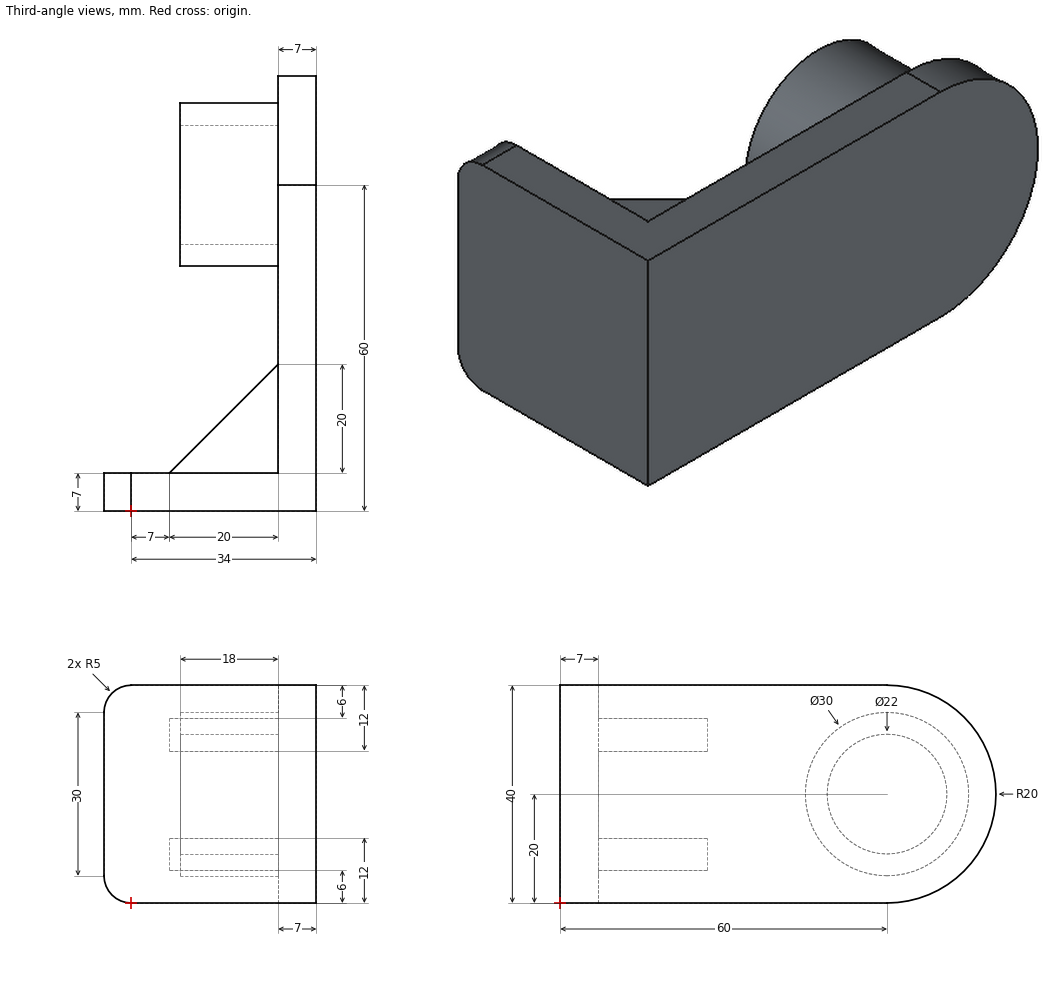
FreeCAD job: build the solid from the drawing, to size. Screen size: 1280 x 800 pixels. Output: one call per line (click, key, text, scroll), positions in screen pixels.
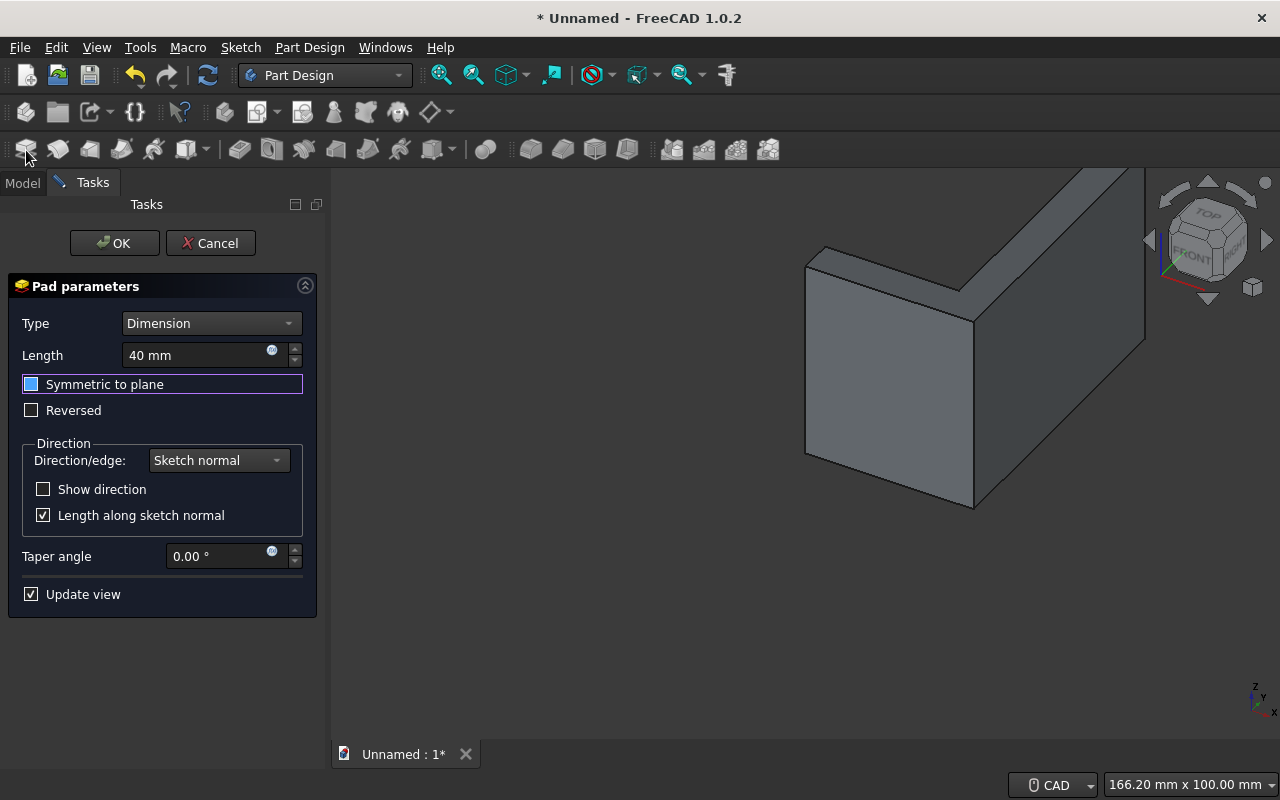
click(115, 243)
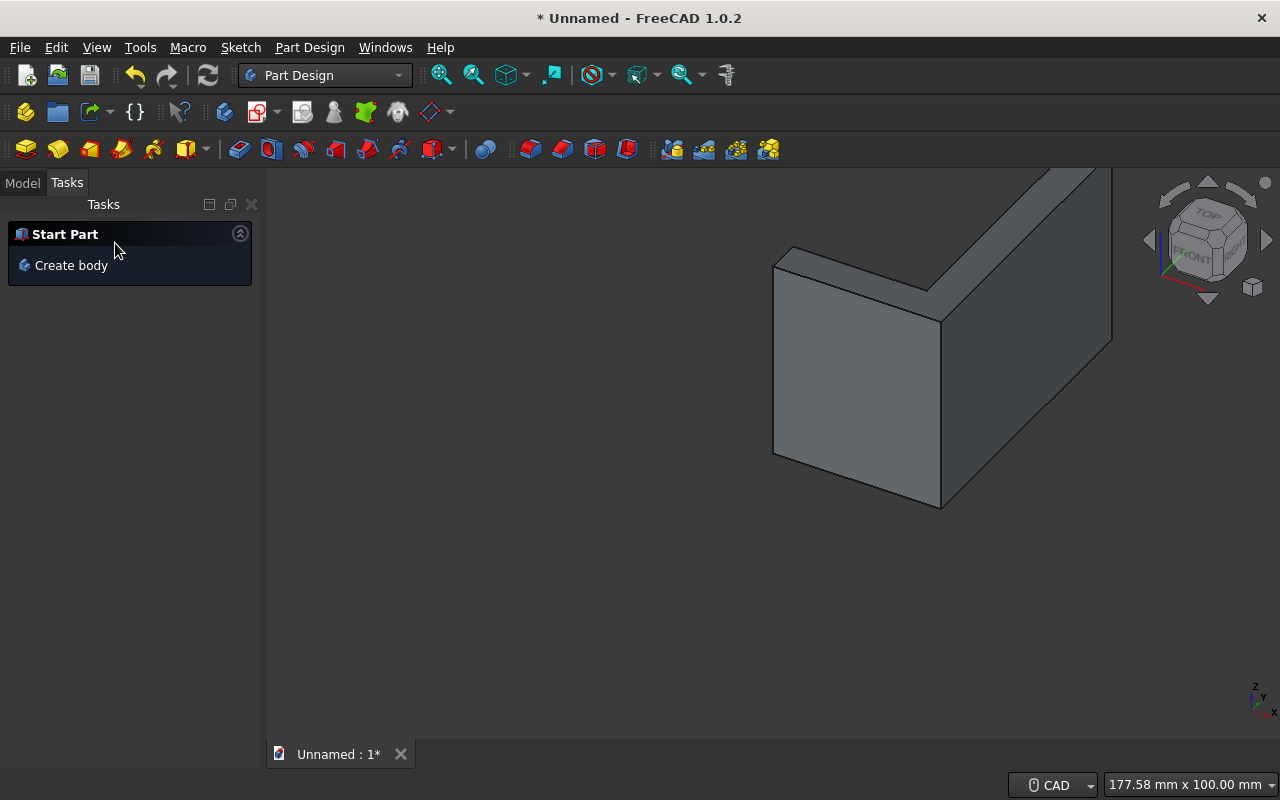
click(442, 76)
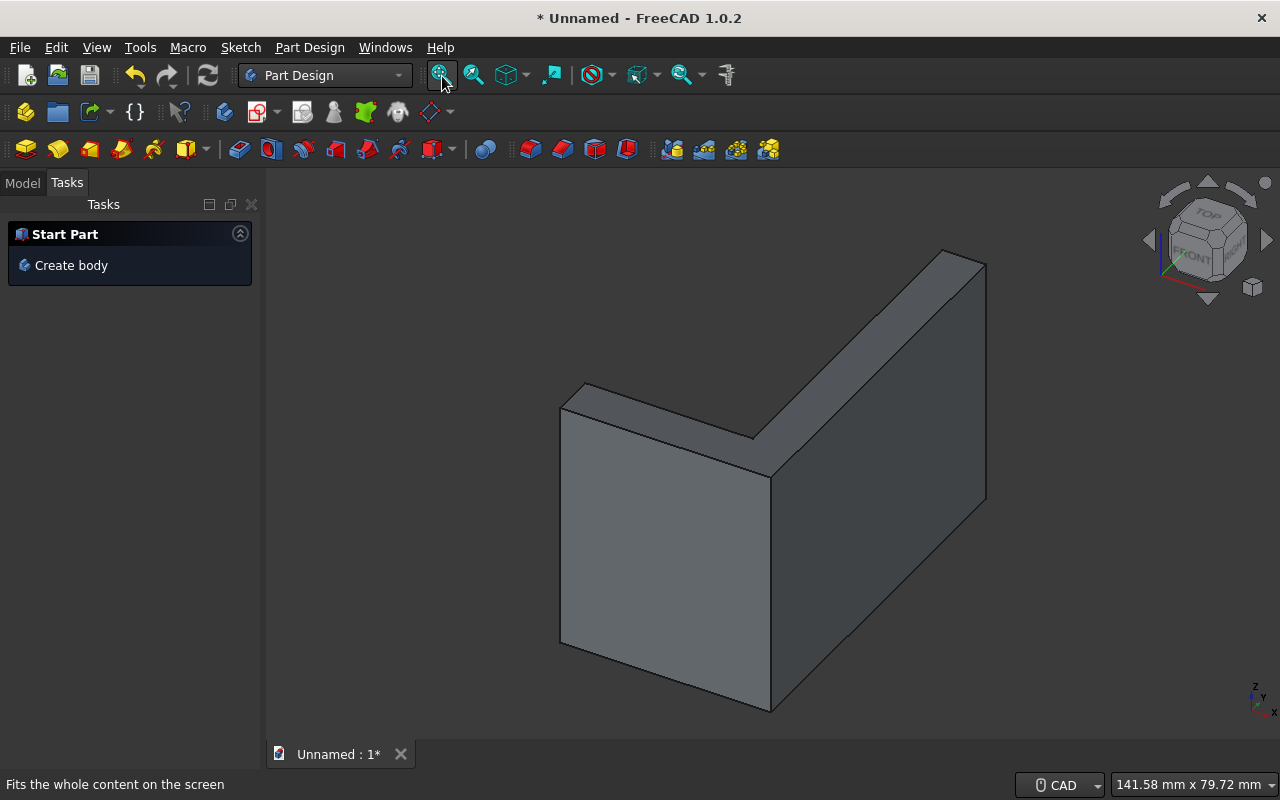
key(4)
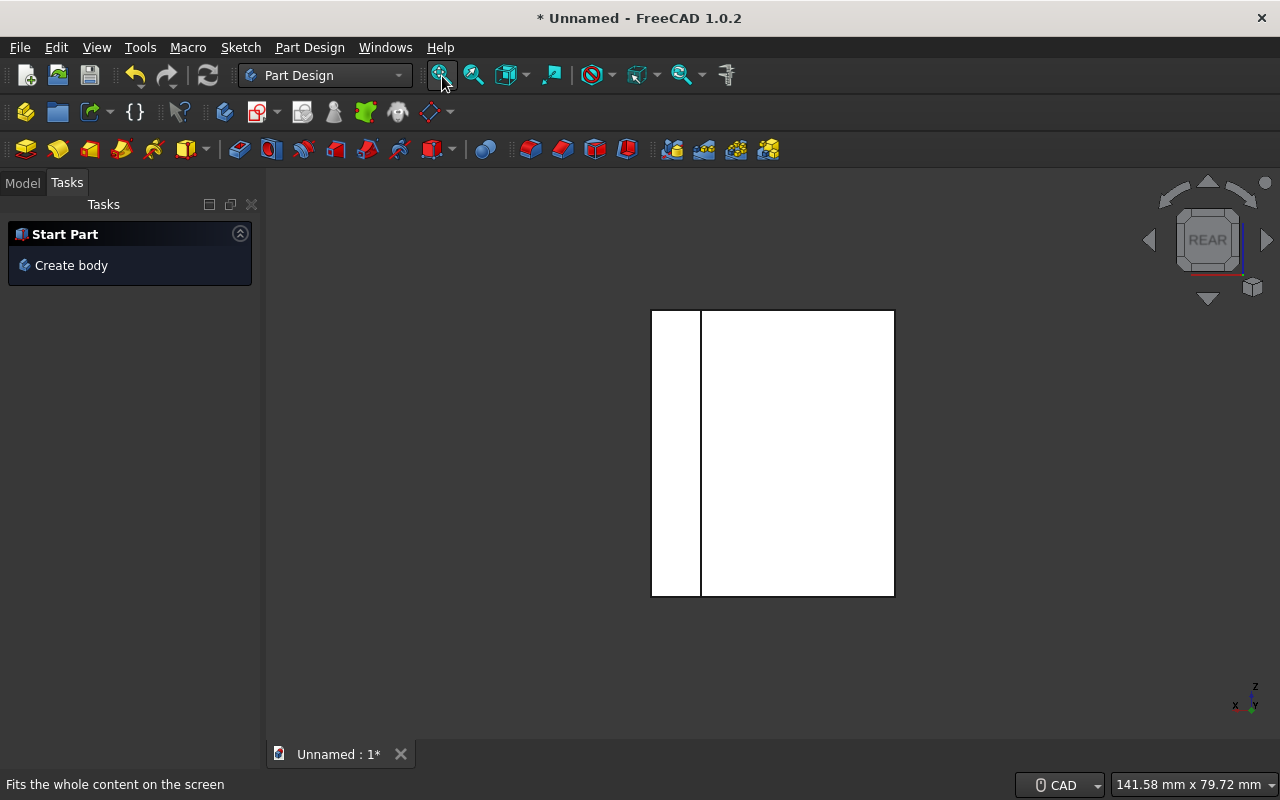
click(798, 412)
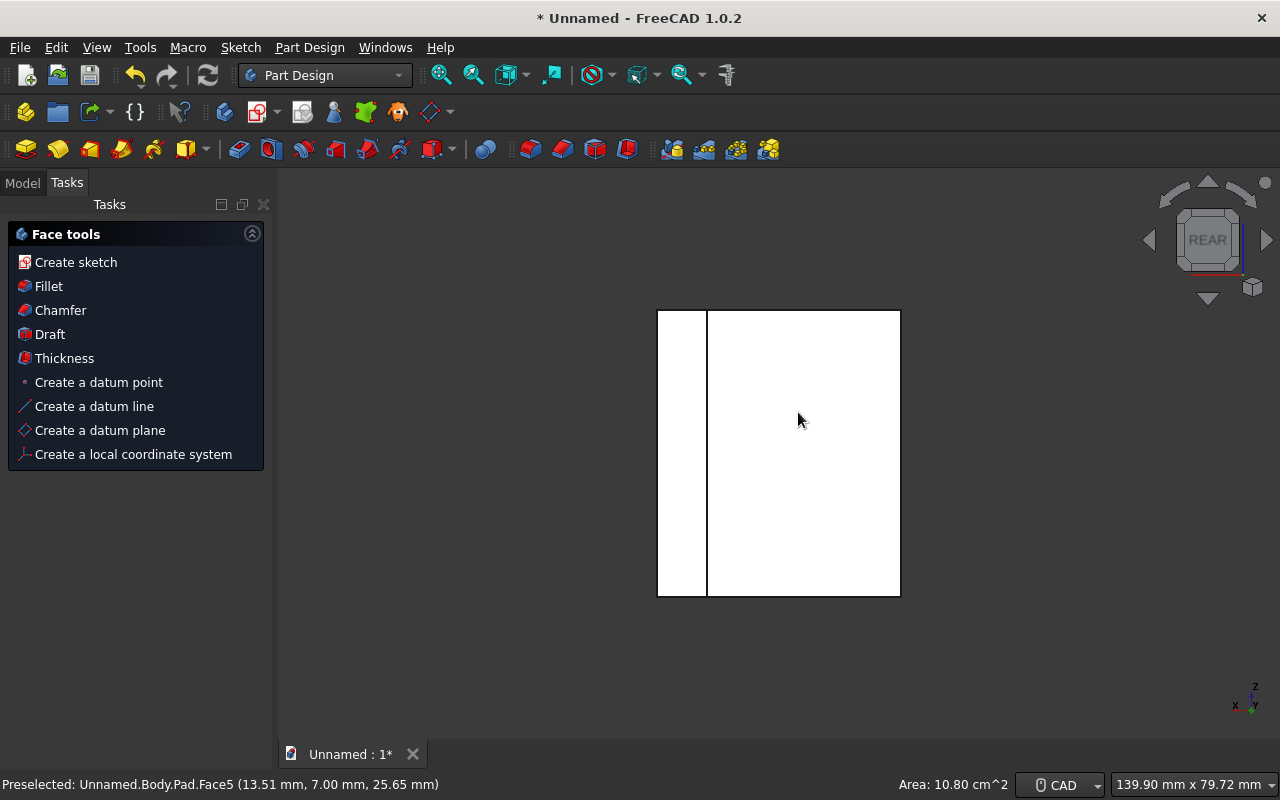
click(258, 112)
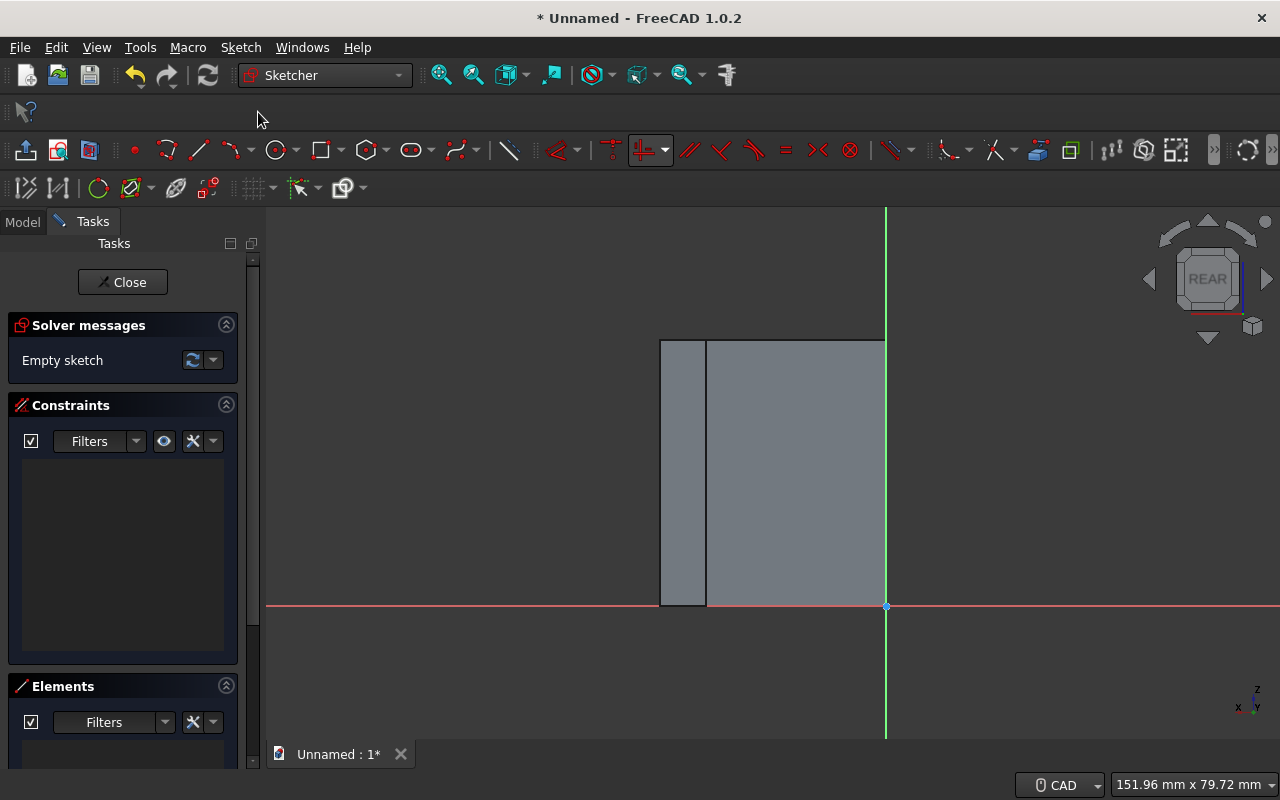
click(200, 150)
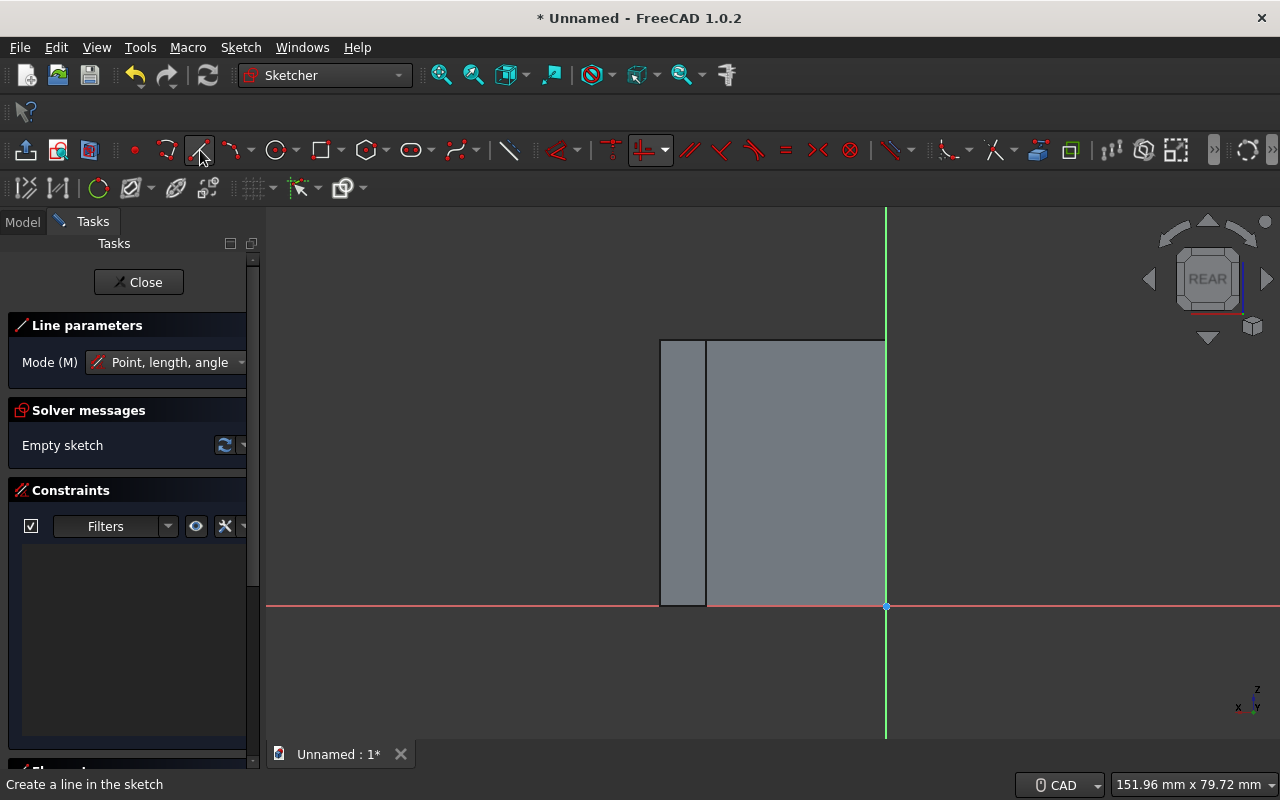
click(920, 573)
click(920, 373)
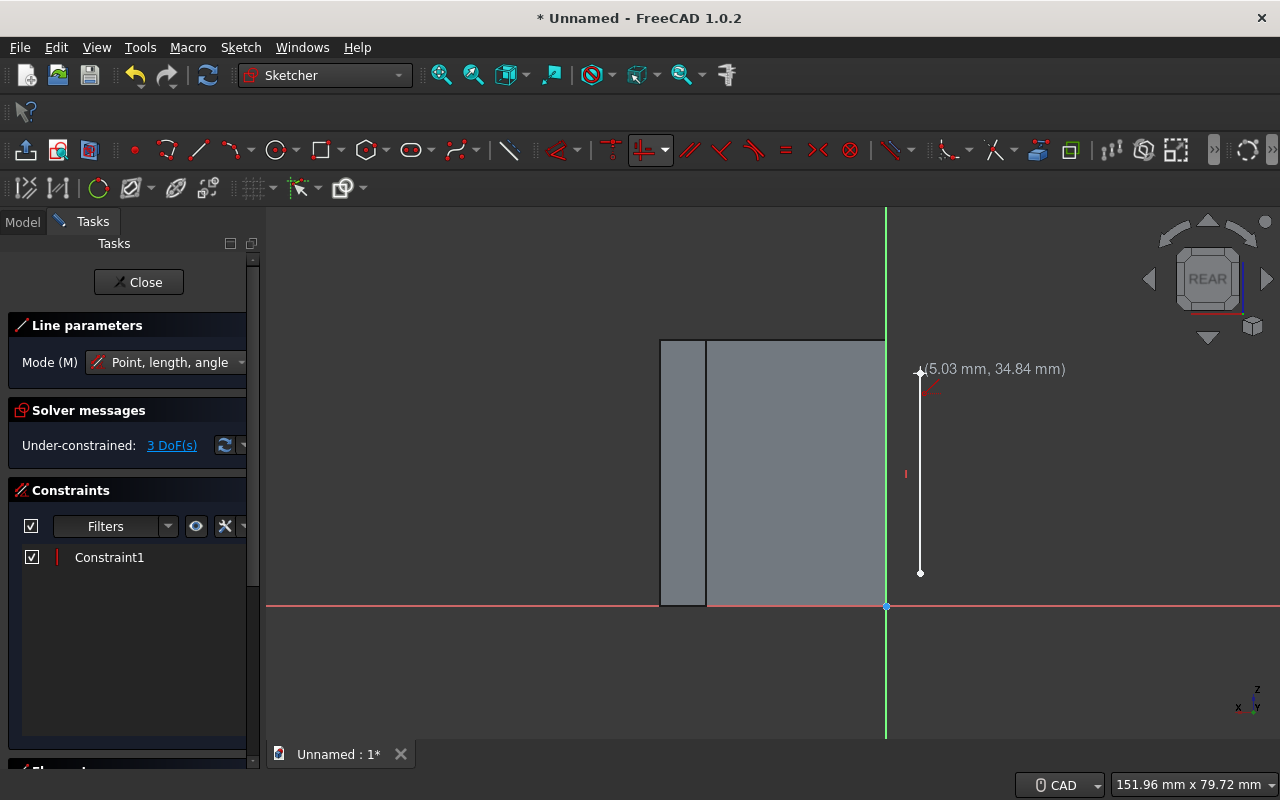
click(886, 340)
click(886, 606)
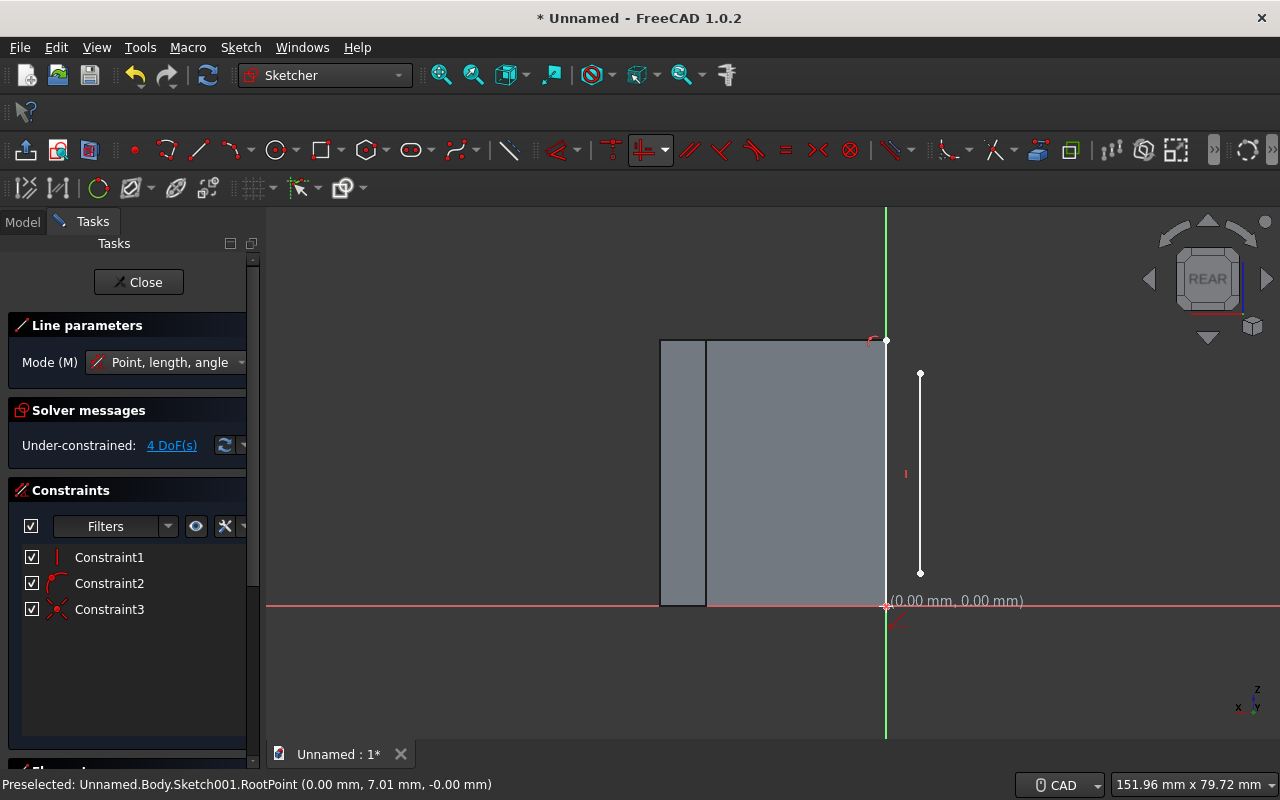
click(232, 150)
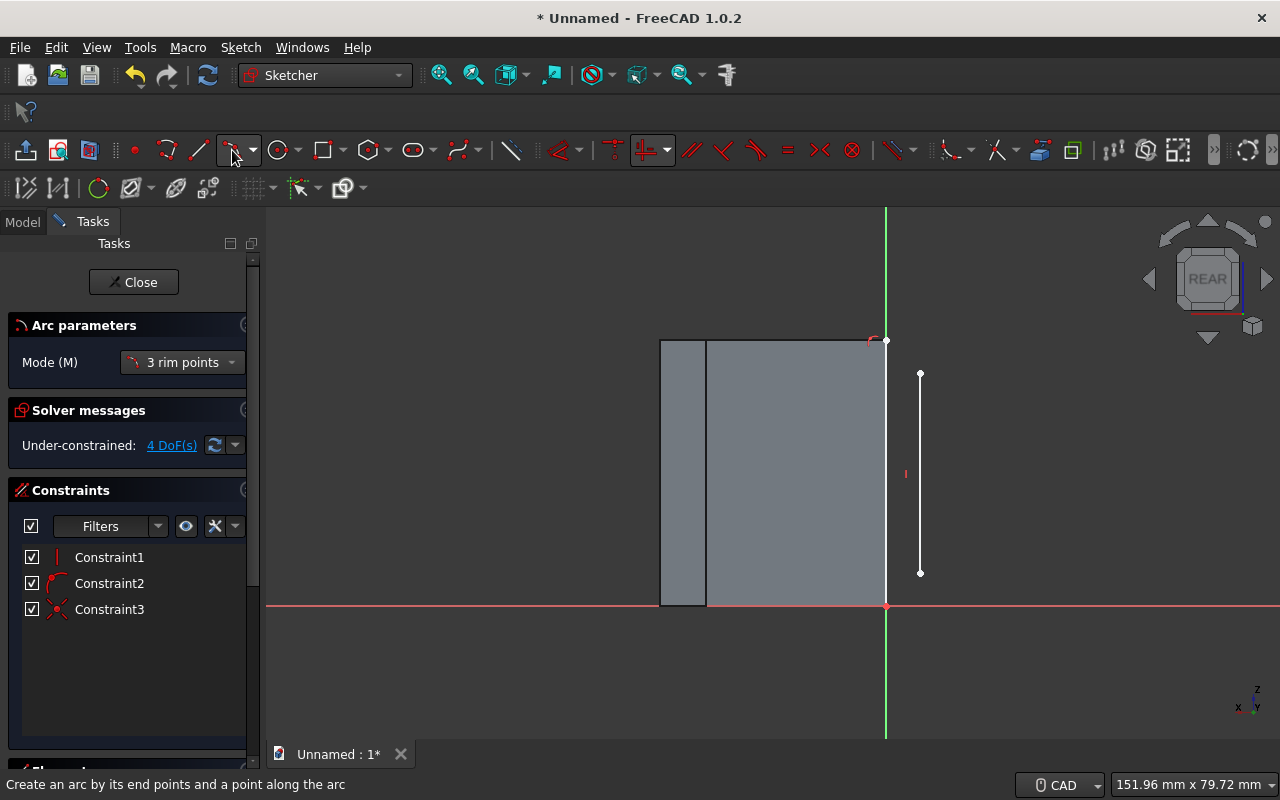
click(920, 374)
click(886, 341)